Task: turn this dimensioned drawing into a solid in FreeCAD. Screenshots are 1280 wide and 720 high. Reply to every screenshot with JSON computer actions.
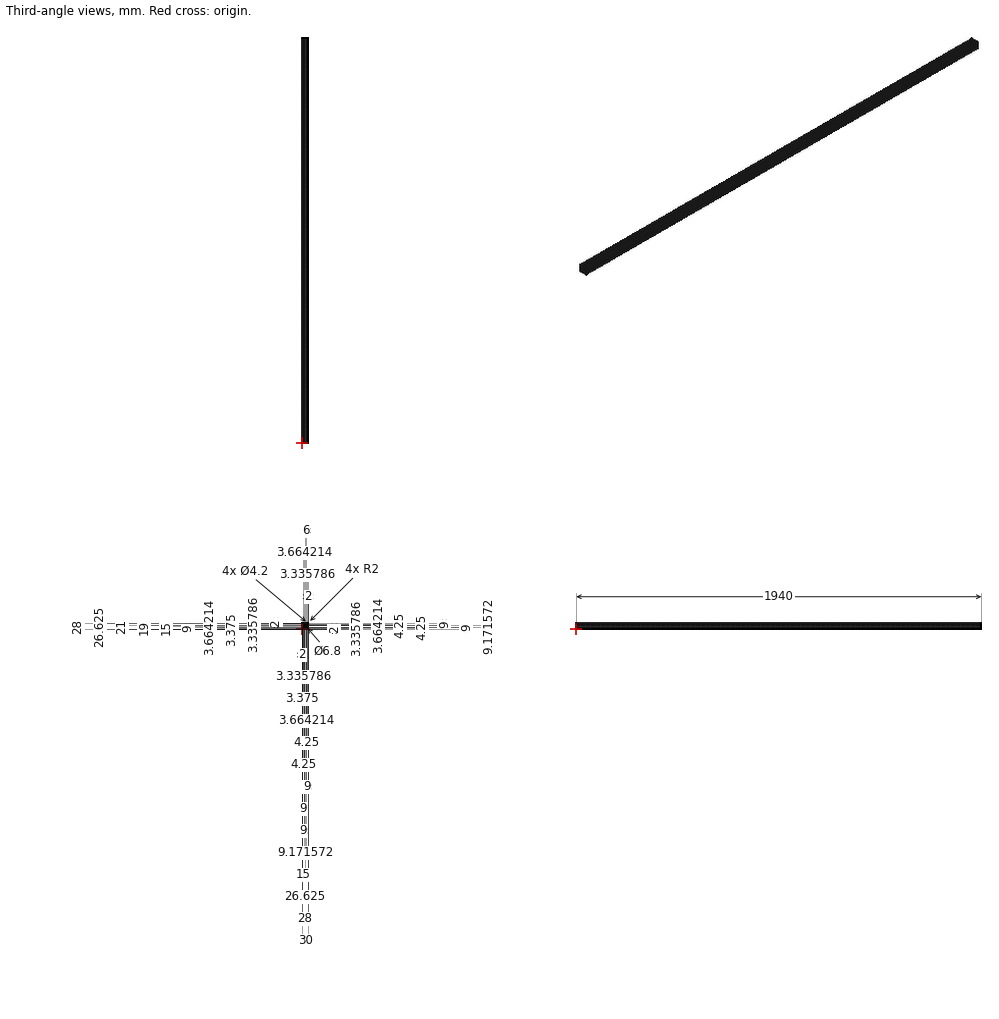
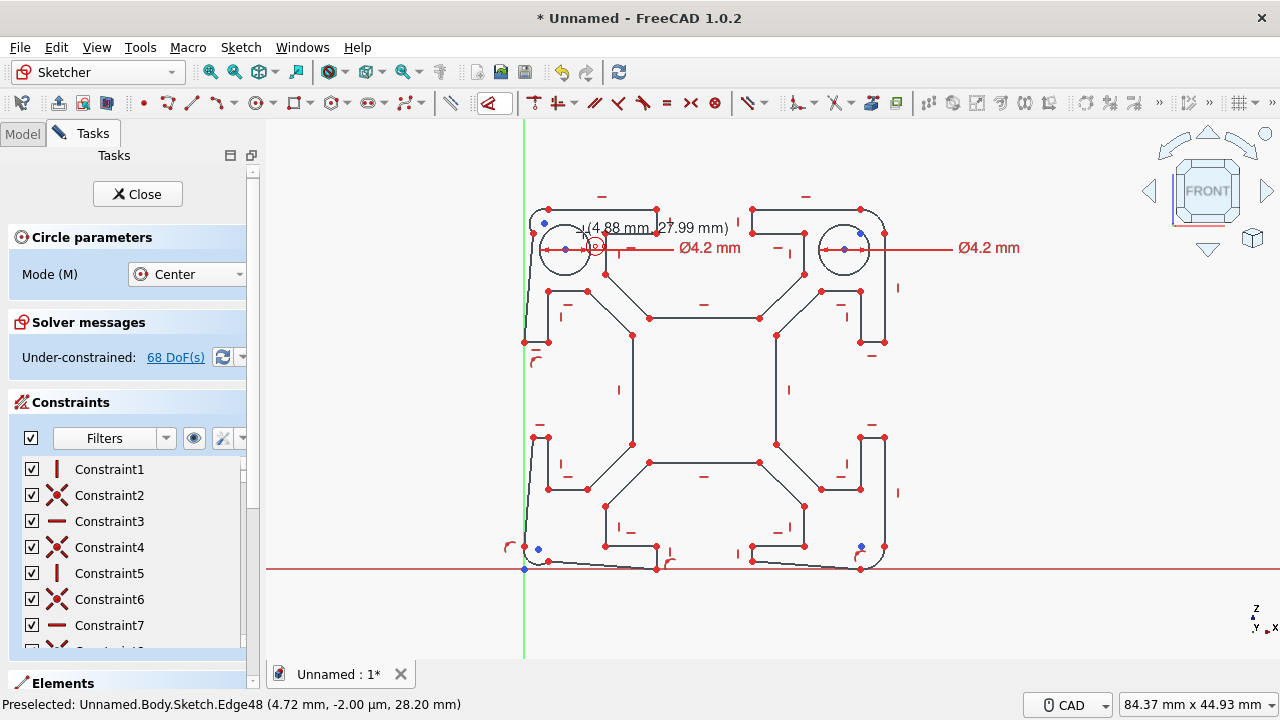
{"action": "left_click", "coordinate": [844, 529]}
{"action": "mouse_move", "coordinate": [862, 511]}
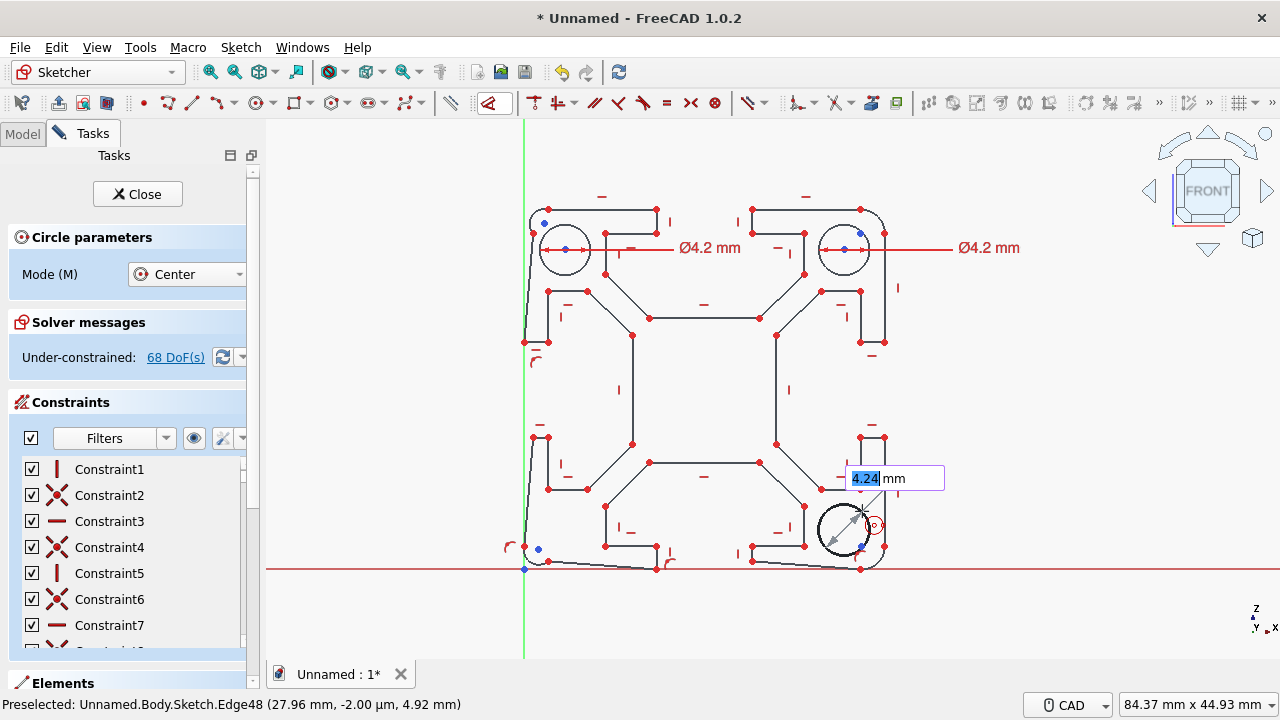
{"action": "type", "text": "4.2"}
{"action": "key", "text": "Return"}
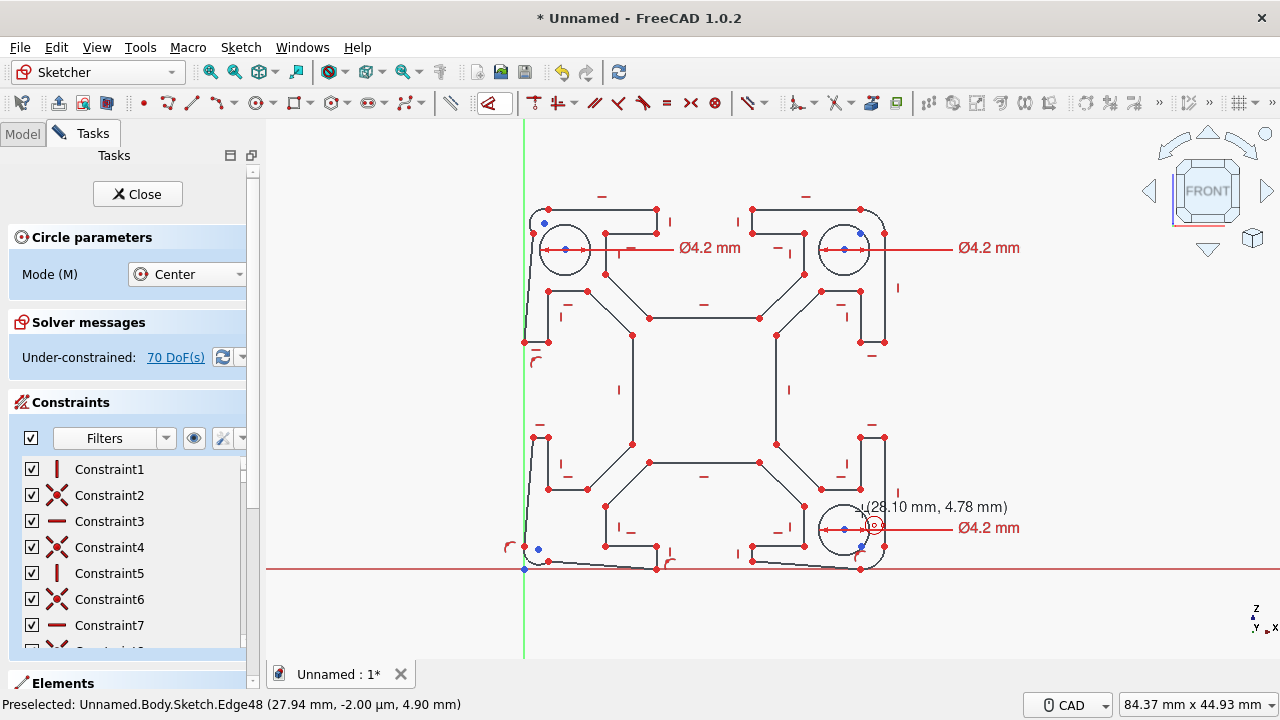
{"action": "left_click", "coordinate": [705, 389]}
{"action": "mouse_move", "coordinate": [733, 360]}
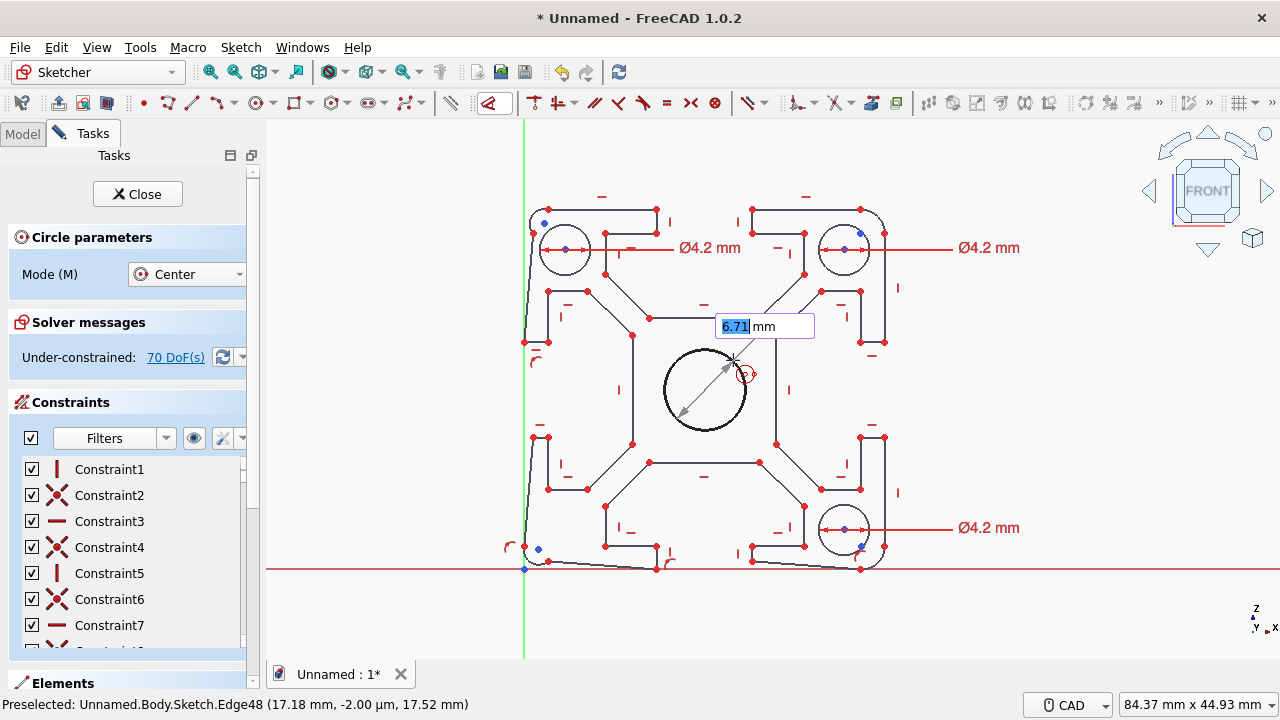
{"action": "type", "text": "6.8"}
{"action": "key", "text": "Return"}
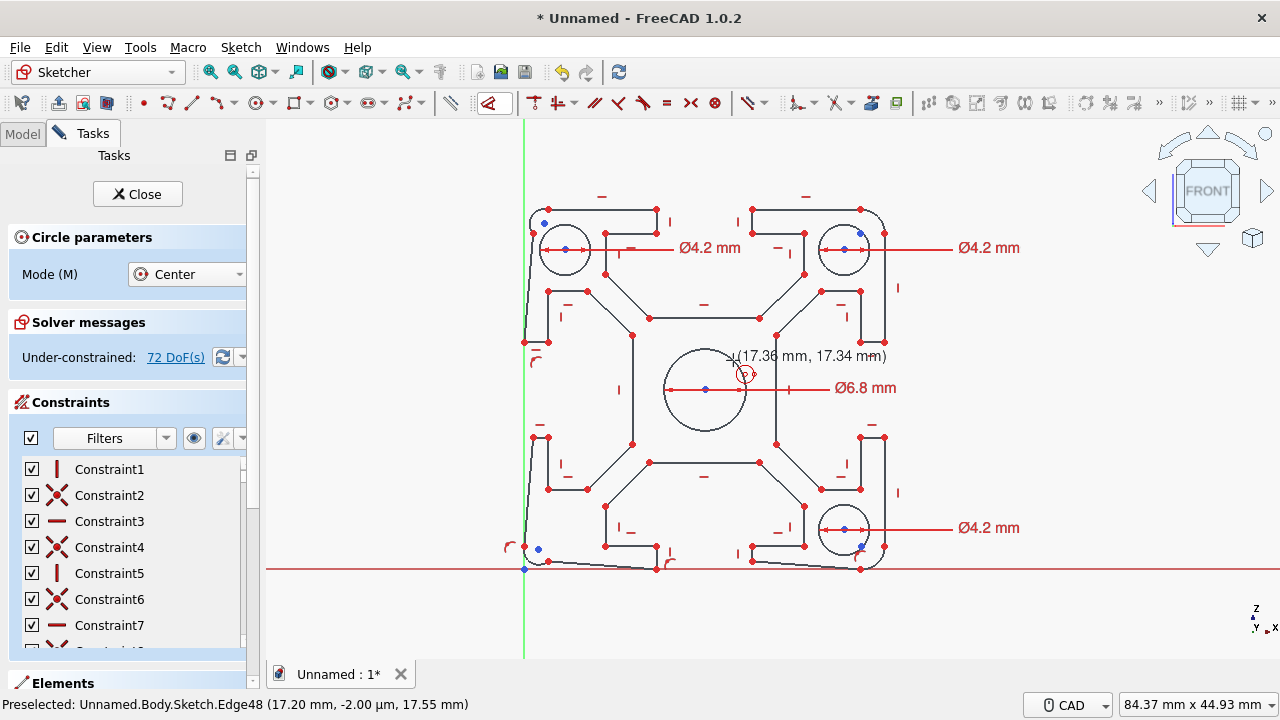
{"action": "left_click", "coordinate": [565, 529]}
{"action": "mouse_move", "coordinate": [583, 511]}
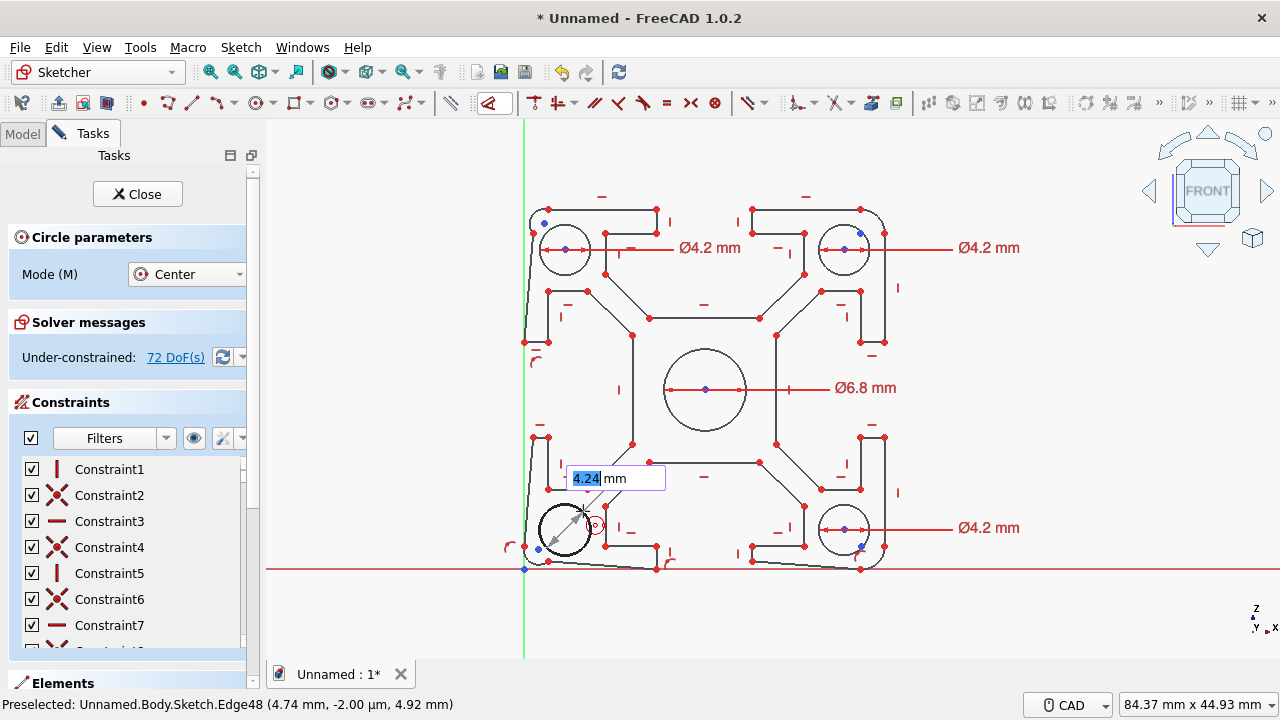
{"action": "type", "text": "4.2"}
{"action": "key", "text": "Return"}
{"action": "key", "text": "Escape"}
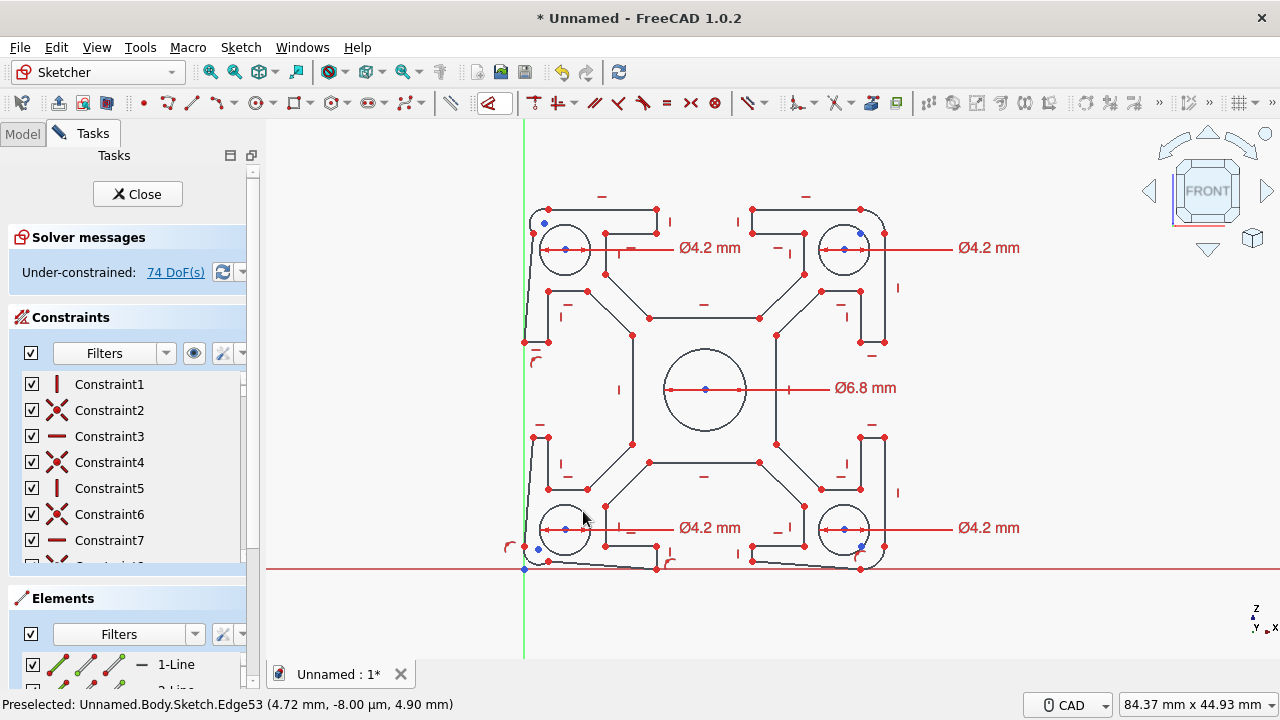
{"action": "left_click", "coordinate": [885, 266]}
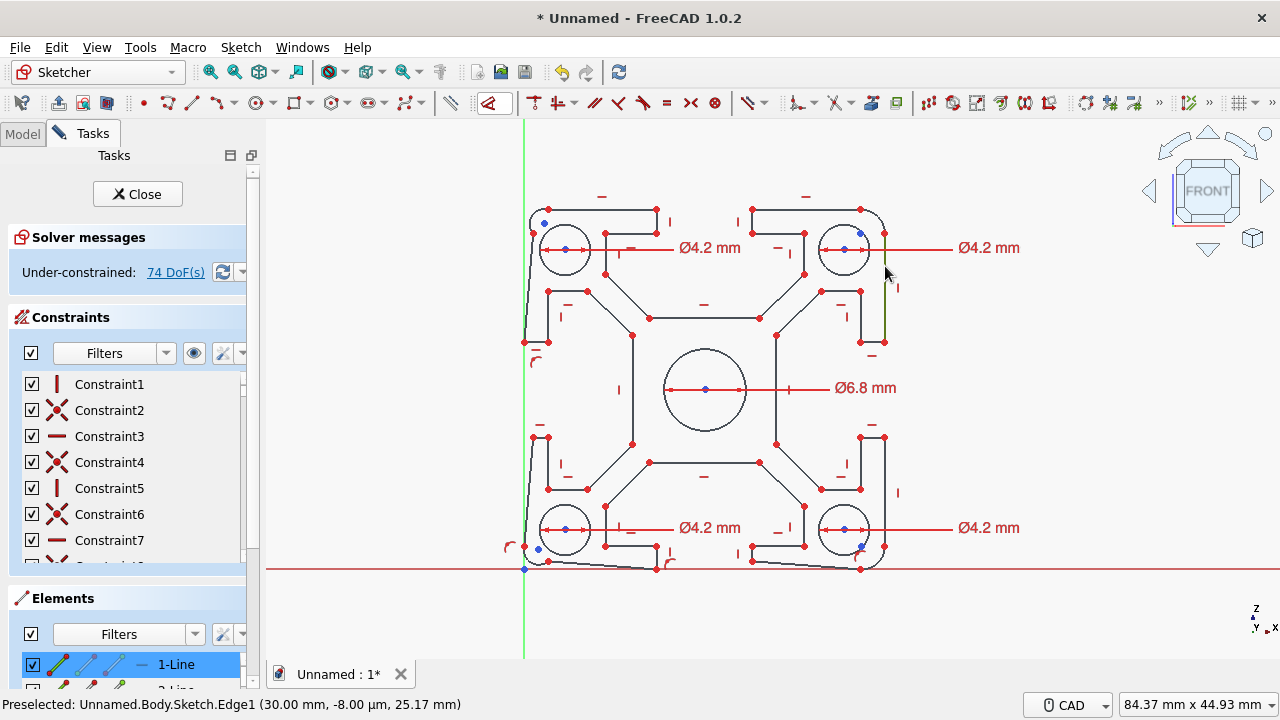
{"action": "scroll", "coordinate": [882, 223], "scroll_direction": "up", "scroll_amount": 2}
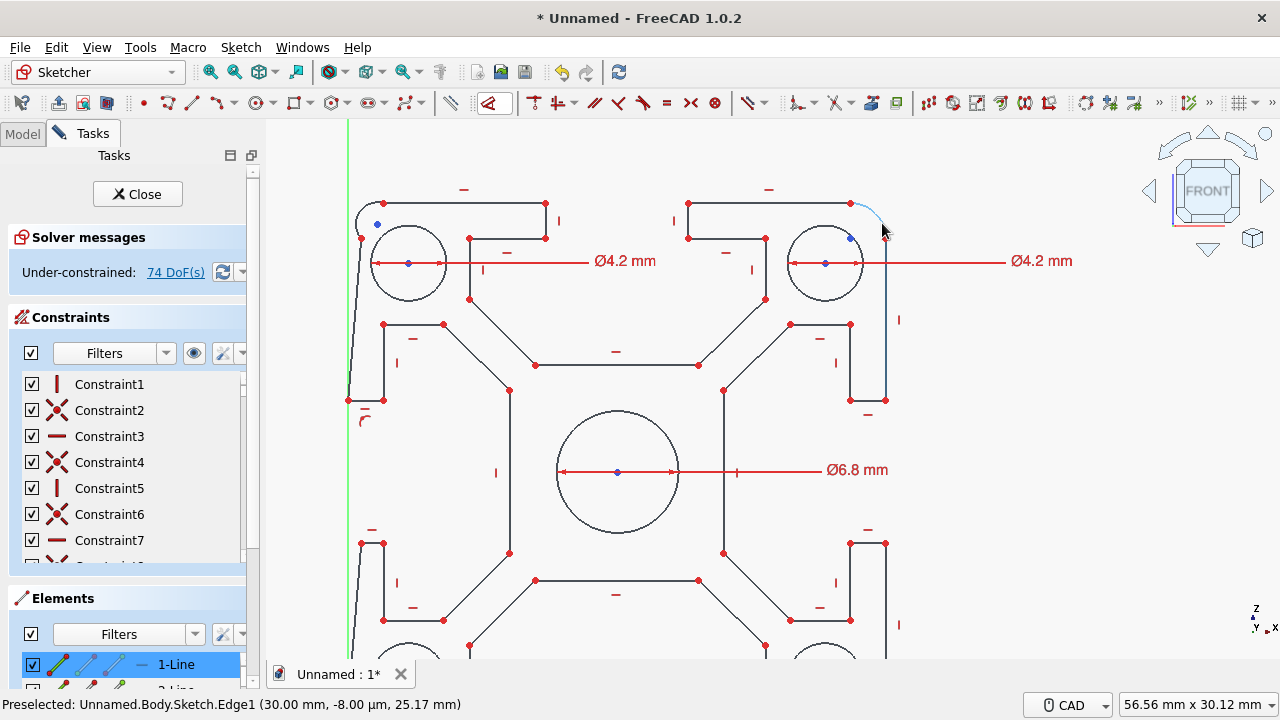
{"action": "left_click", "coordinate": [882, 222]}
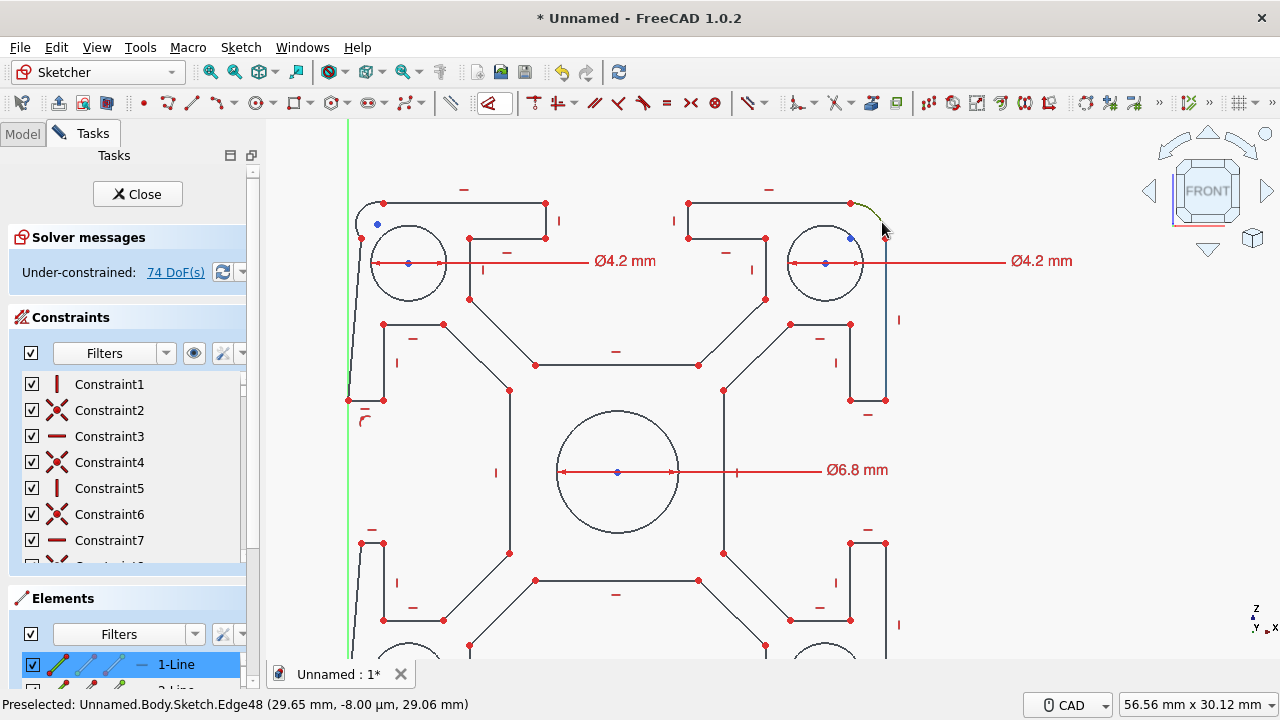
{"action": "key", "text": "t"}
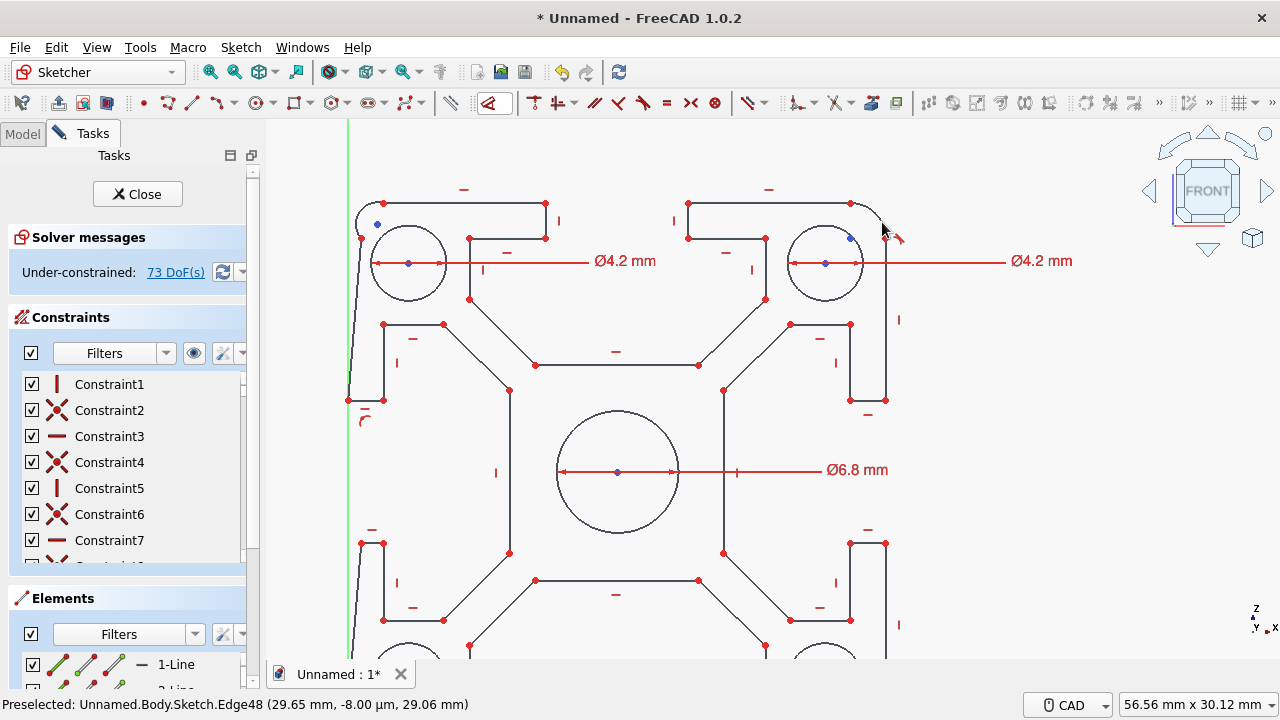
{"action": "left_click", "coordinate": [886, 592]}